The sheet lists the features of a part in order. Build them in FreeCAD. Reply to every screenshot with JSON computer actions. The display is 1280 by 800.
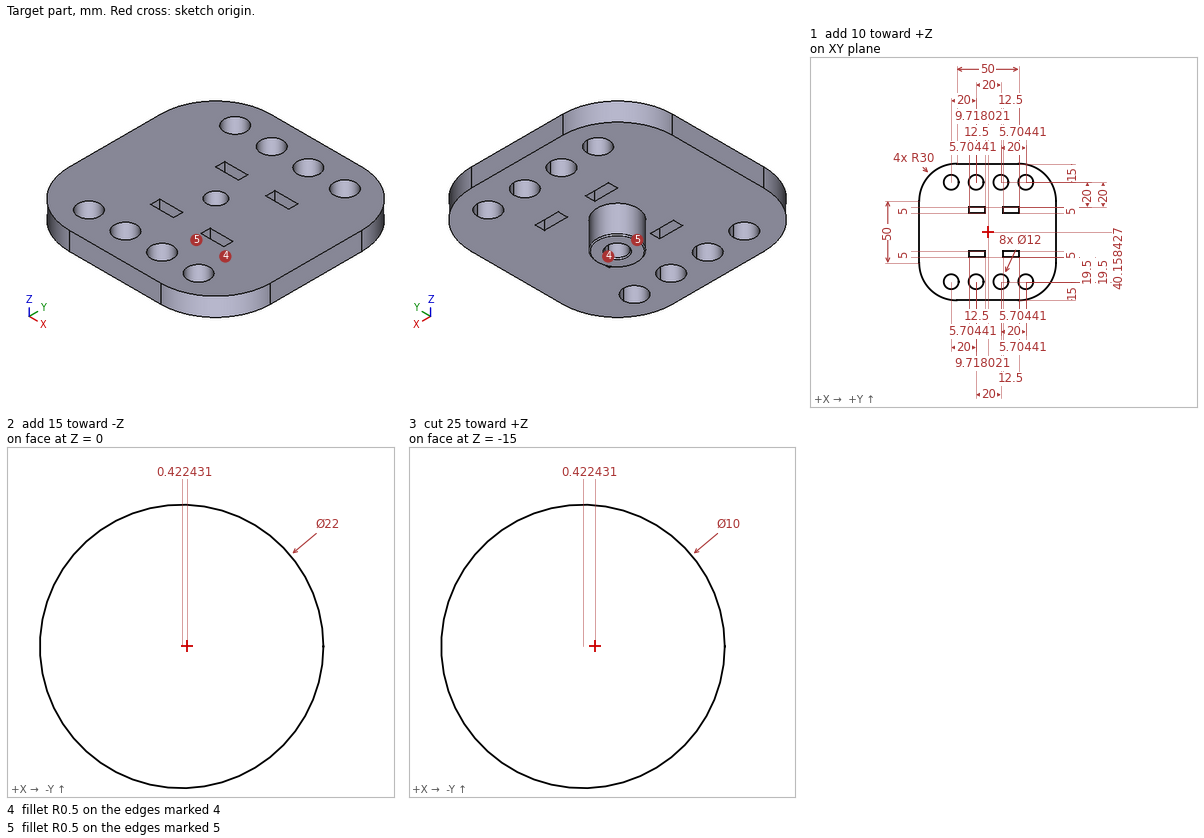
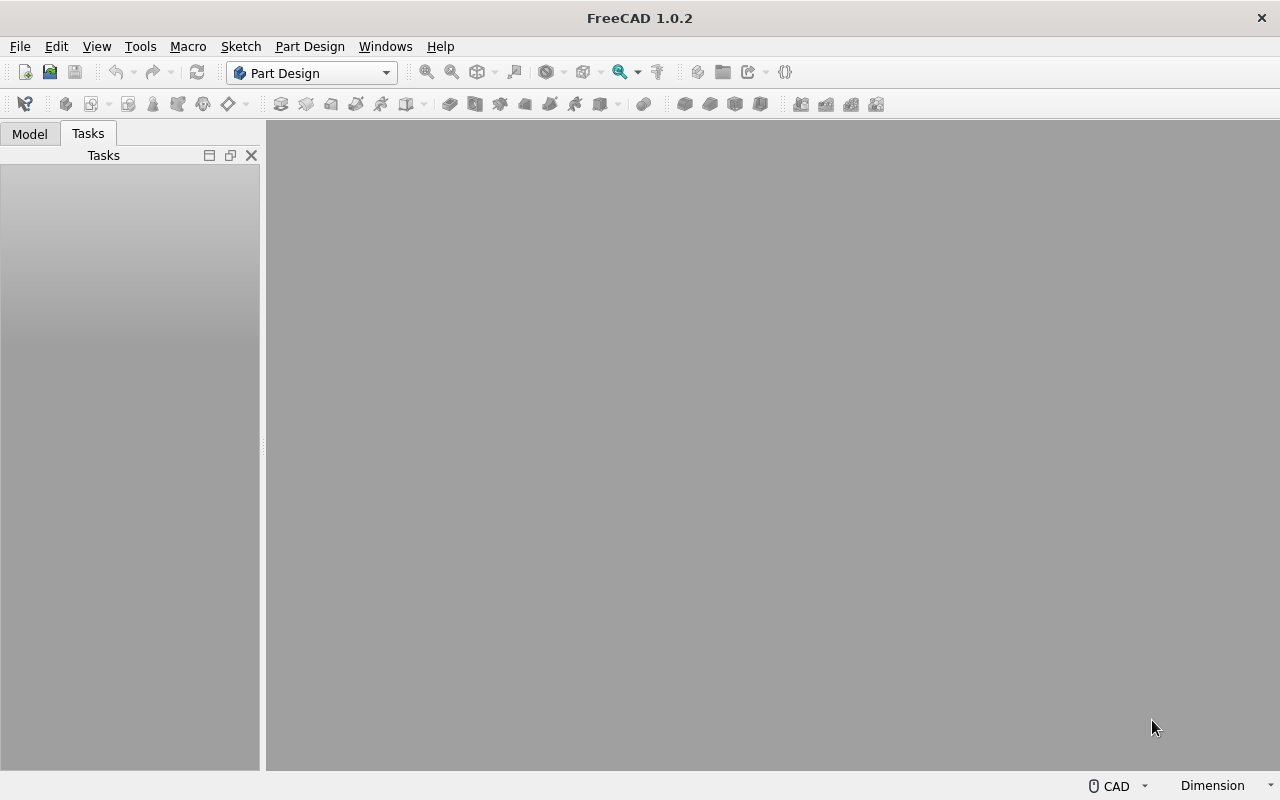
{"action": "left_click", "coordinate": [25, 72]}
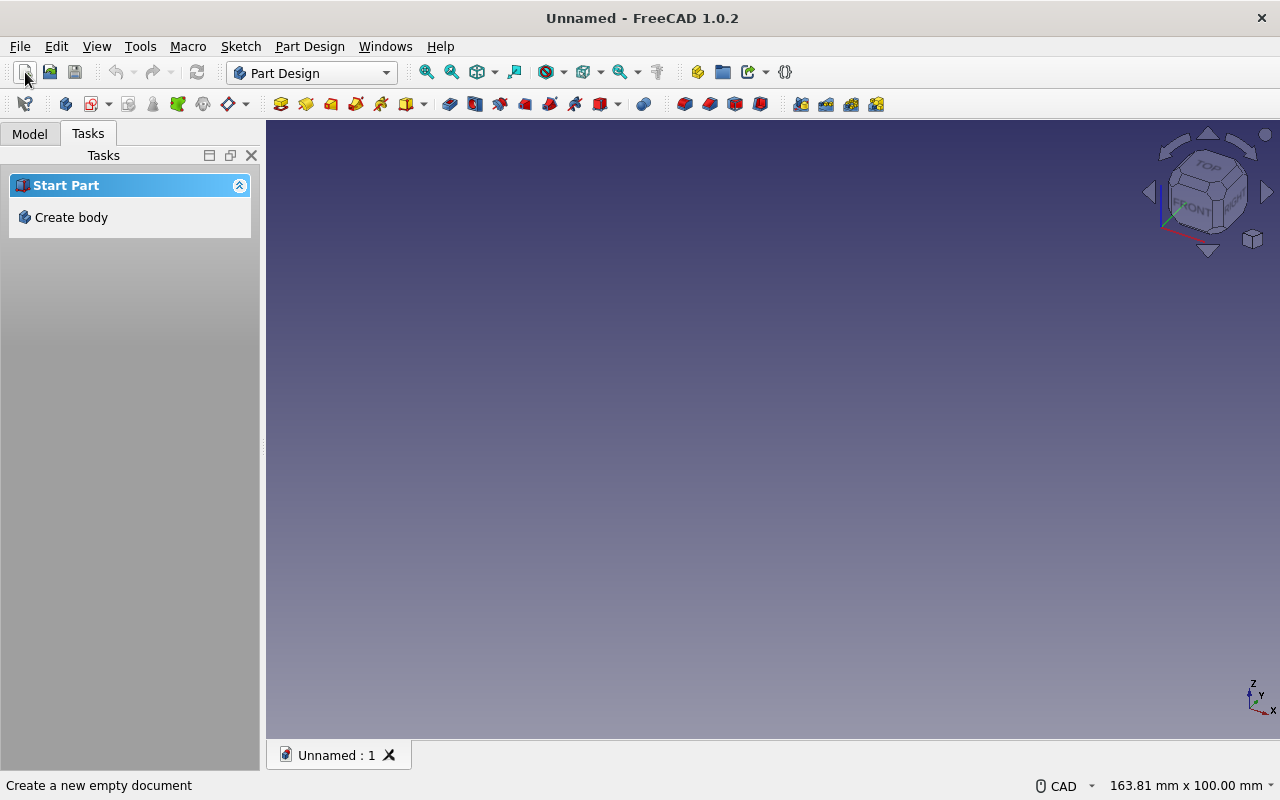
{"action": "left_click", "coordinate": [90, 104]}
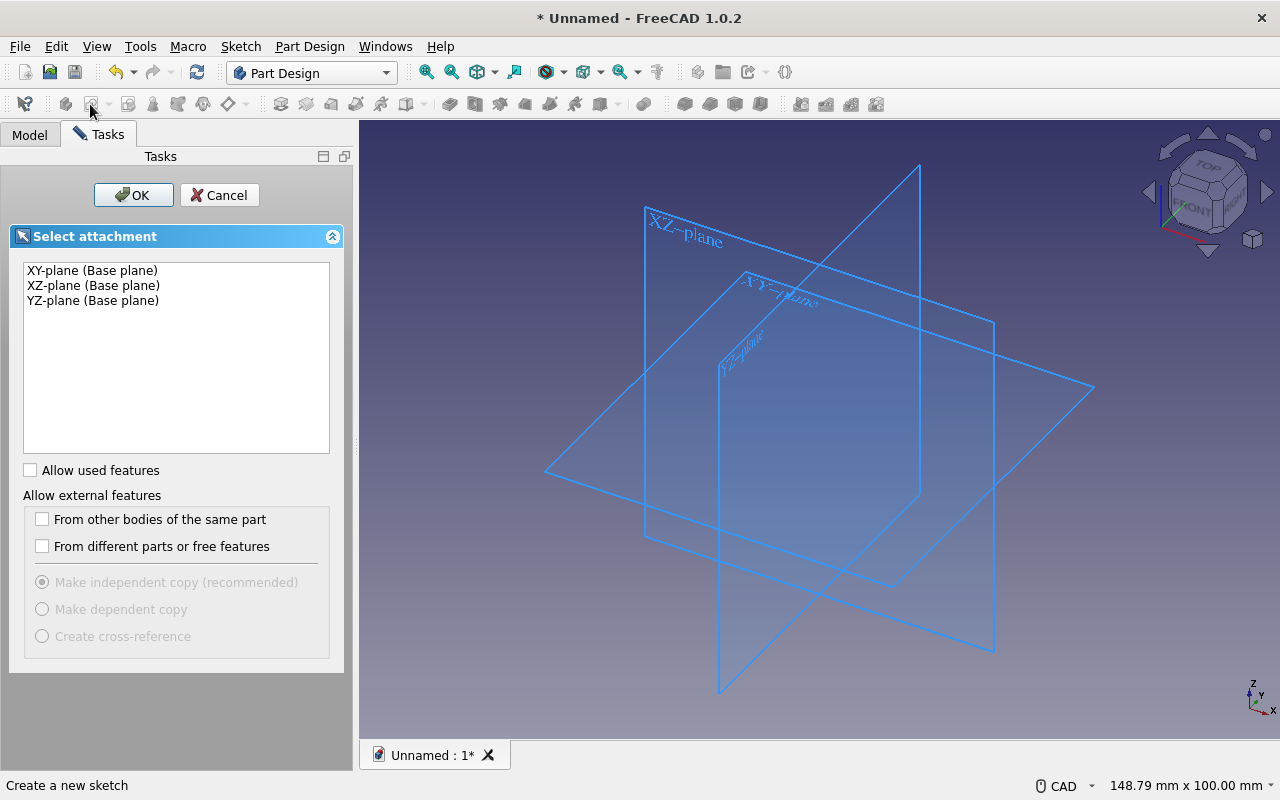
{"action": "left_click", "coordinate": [84, 270]}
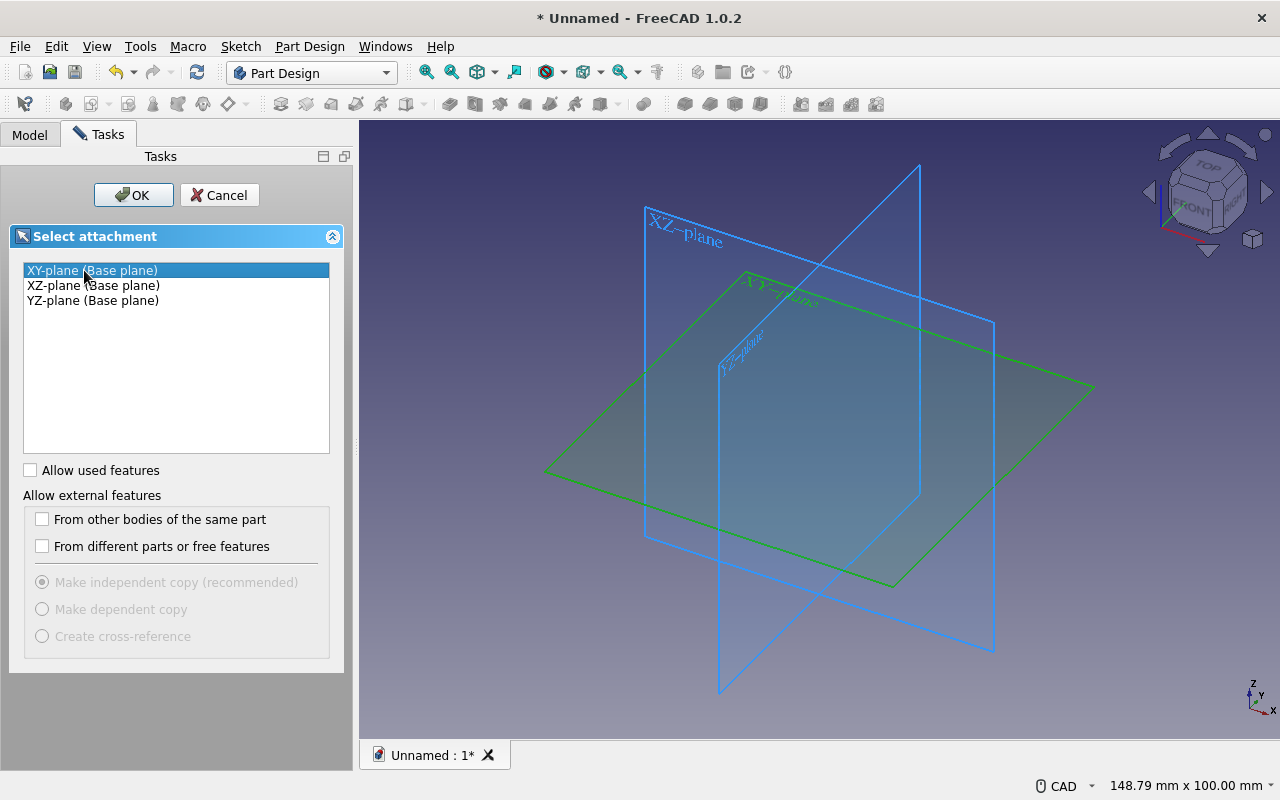
{"action": "left_click", "coordinate": [134, 195]}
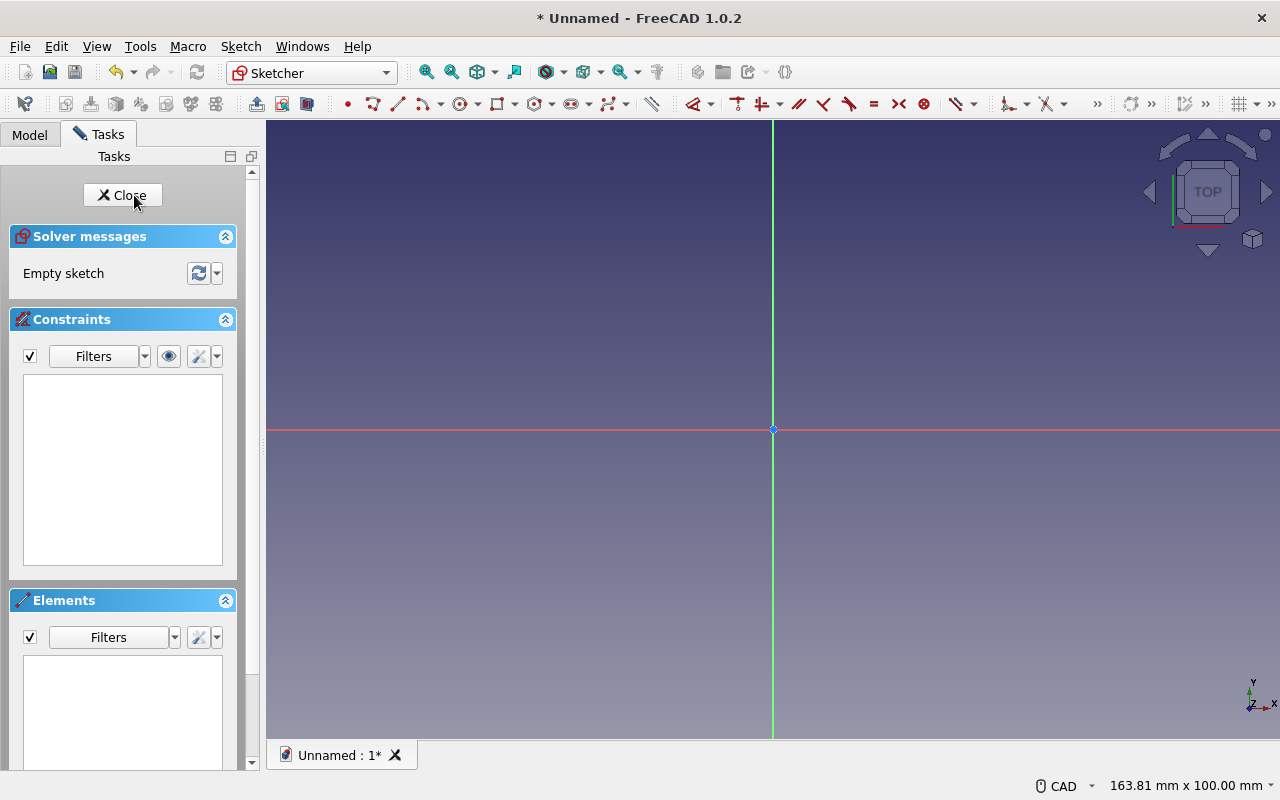
{"action": "scroll", "coordinate": [624, 428], "scroll_direction": "down", "scroll_amount": 3}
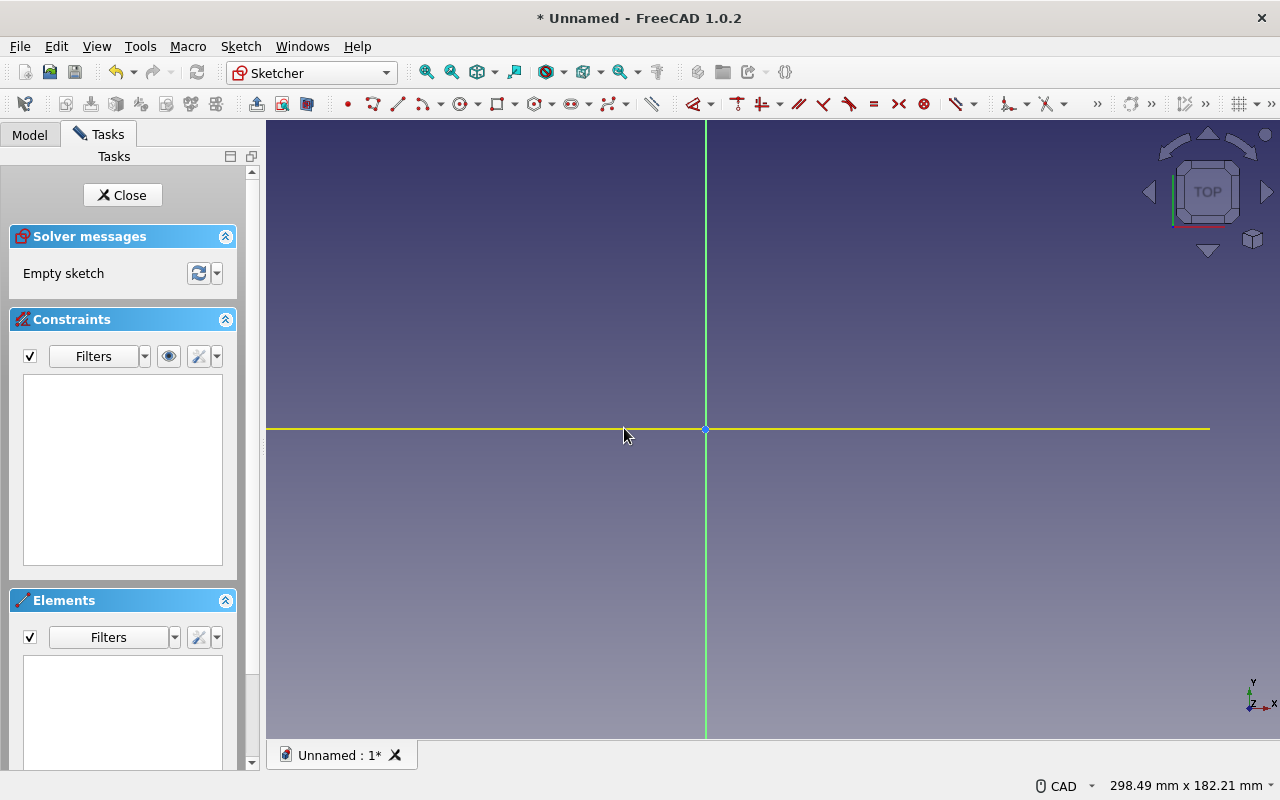
{"action": "key", "text": "g l"}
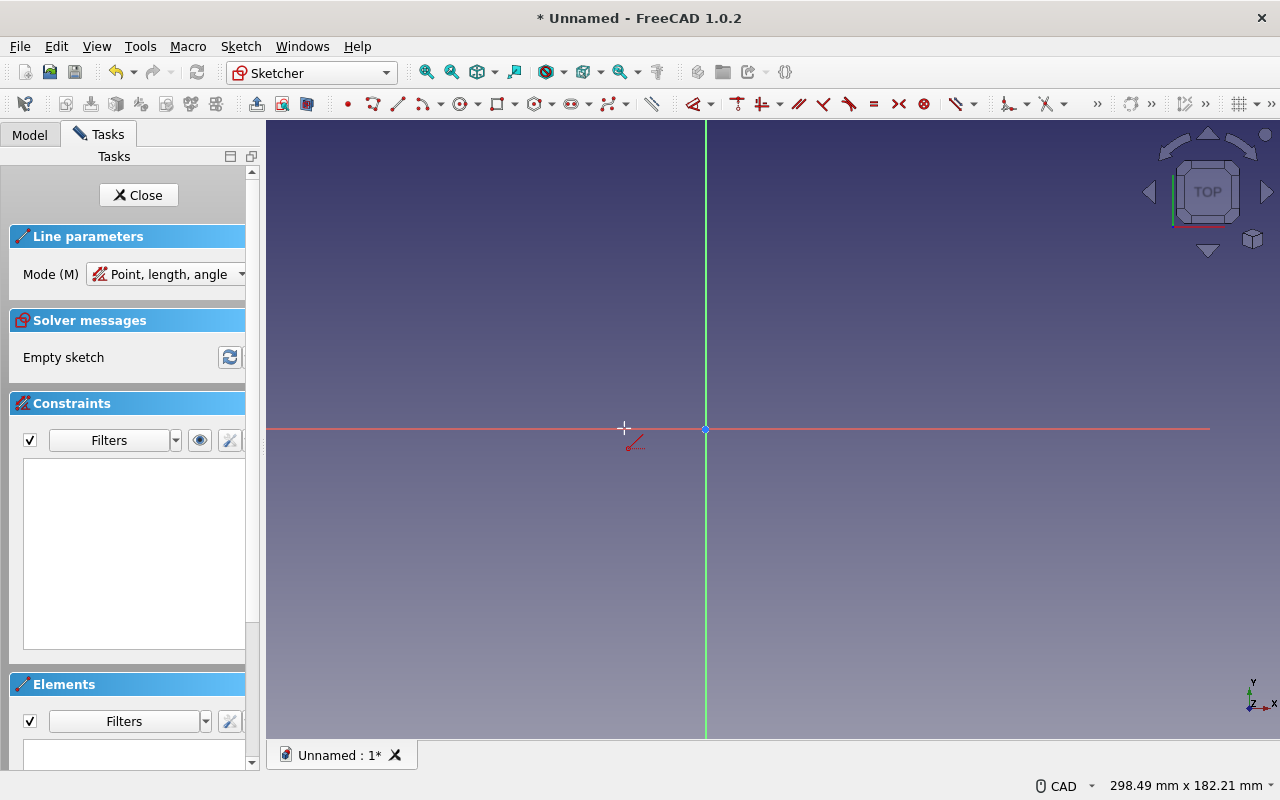
{"action": "left_click", "coordinate": [789, 243]}
{"action": "left_click", "coordinate": [620, 243]}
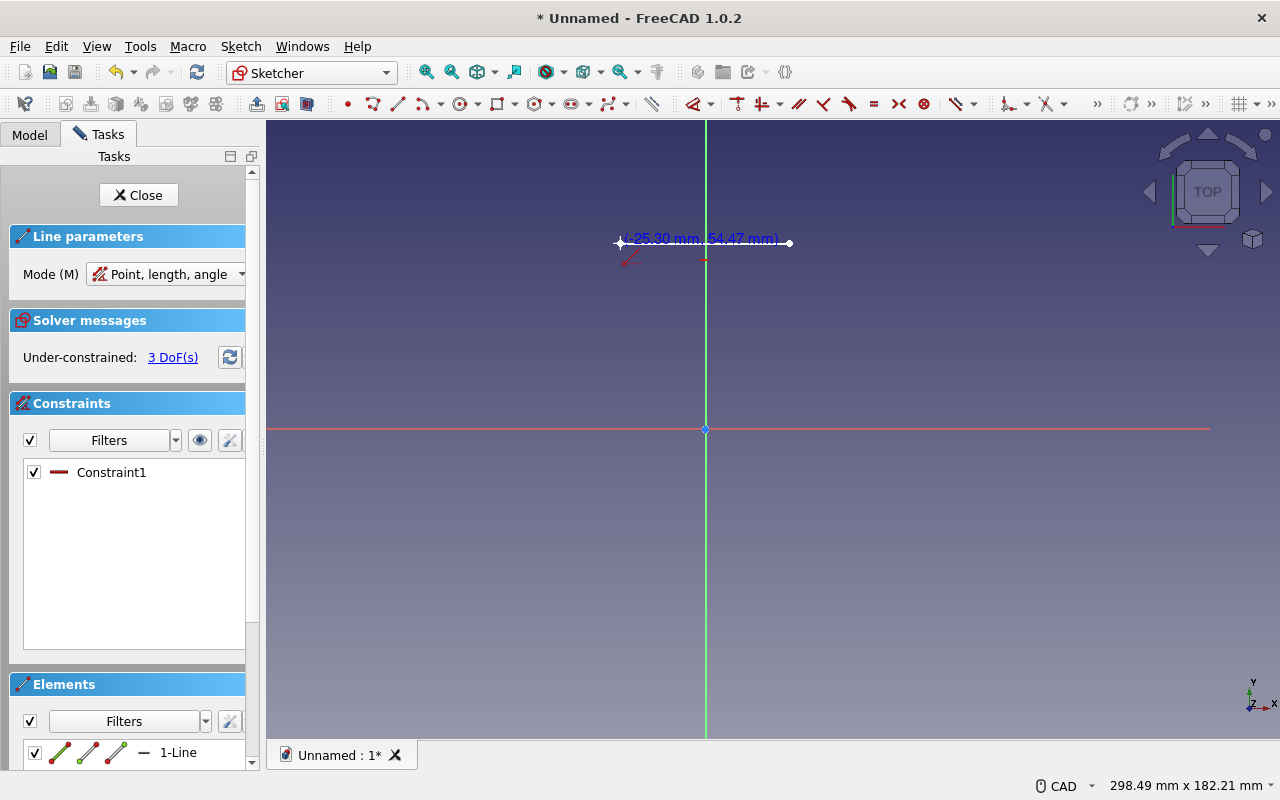
{"action": "left_click", "coordinate": [518, 345]}
{"action": "left_click", "coordinate": [518, 515]}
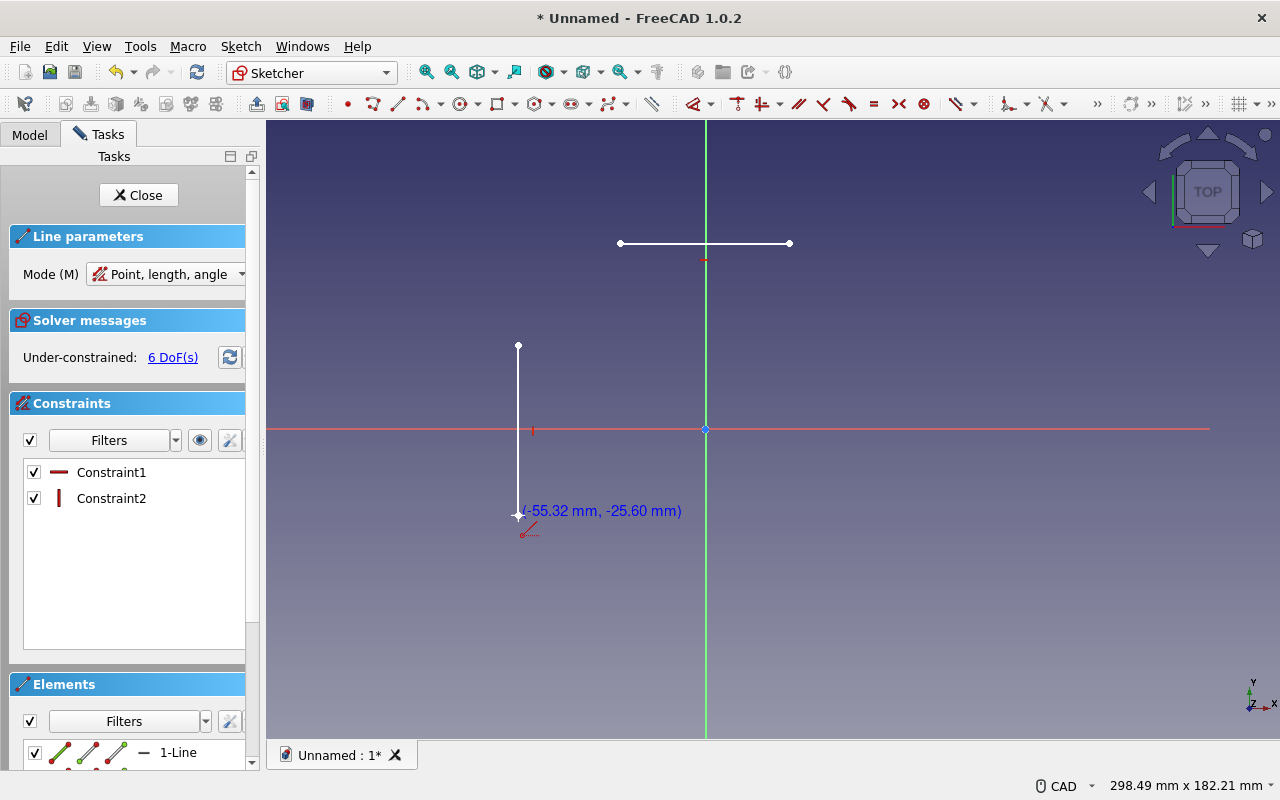
{"action": "left_click", "coordinate": [620, 616]}
{"action": "left_click", "coordinate": [789, 616]}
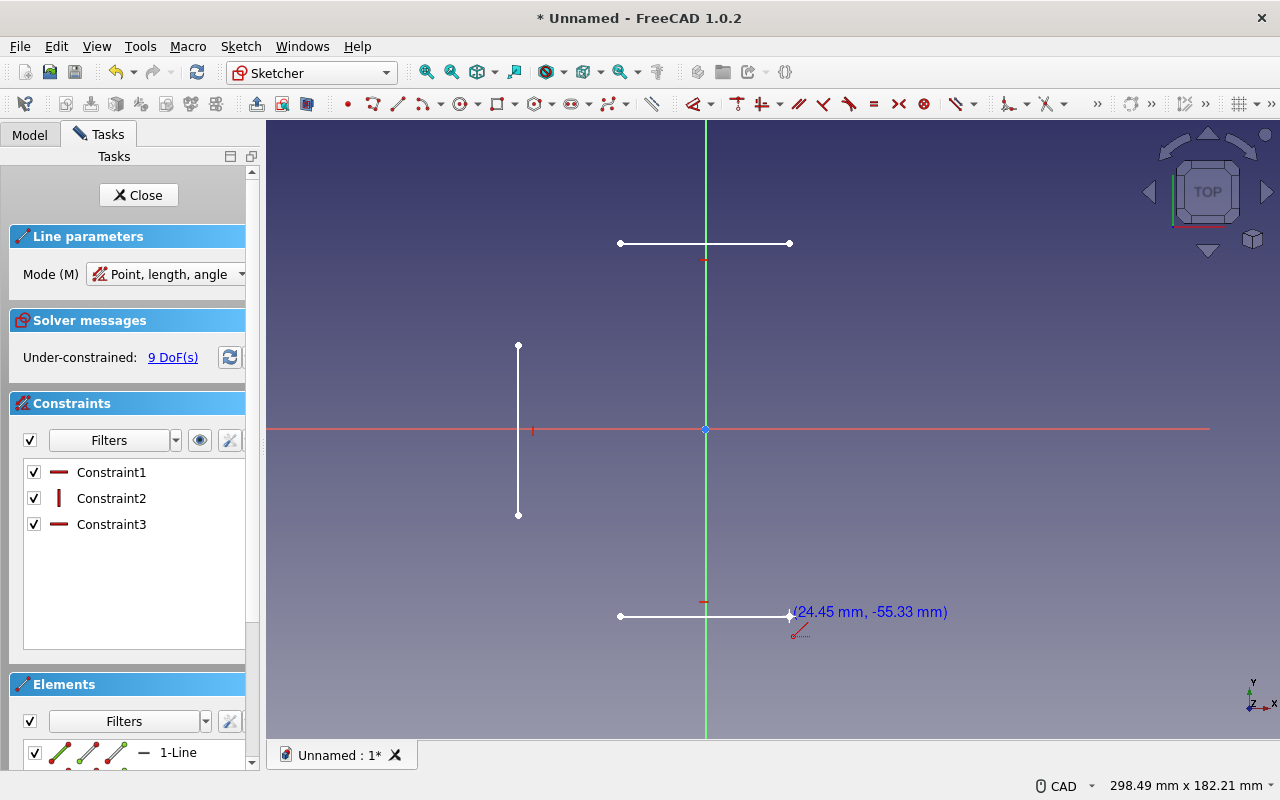
{"action": "left_click", "coordinate": [891, 515]}
{"action": "left_click", "coordinate": [891, 345]}